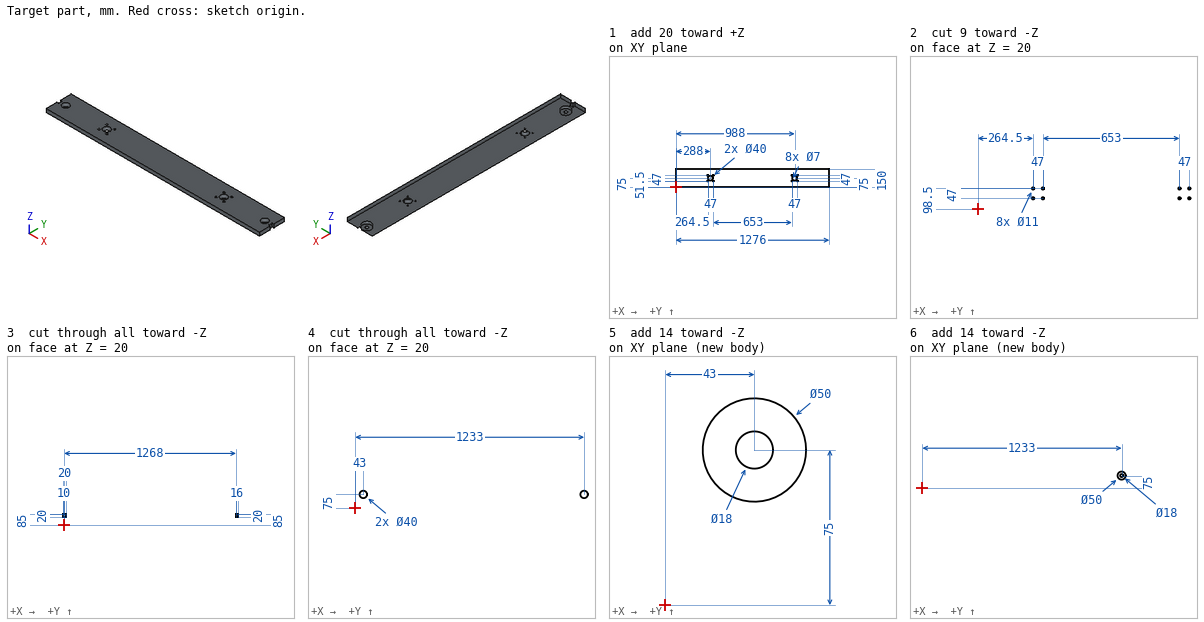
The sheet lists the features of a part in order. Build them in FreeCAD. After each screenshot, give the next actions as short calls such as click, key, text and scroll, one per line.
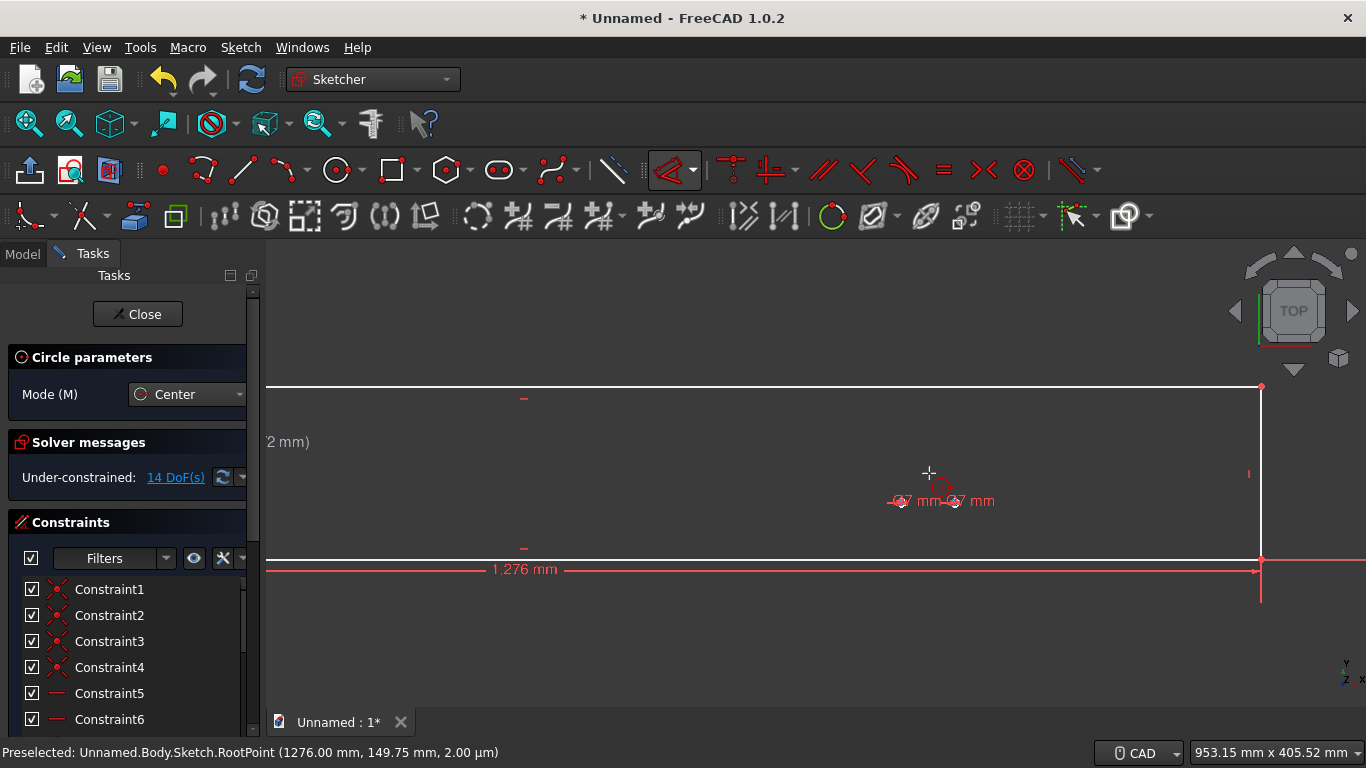
click(929, 473)
move(945, 457)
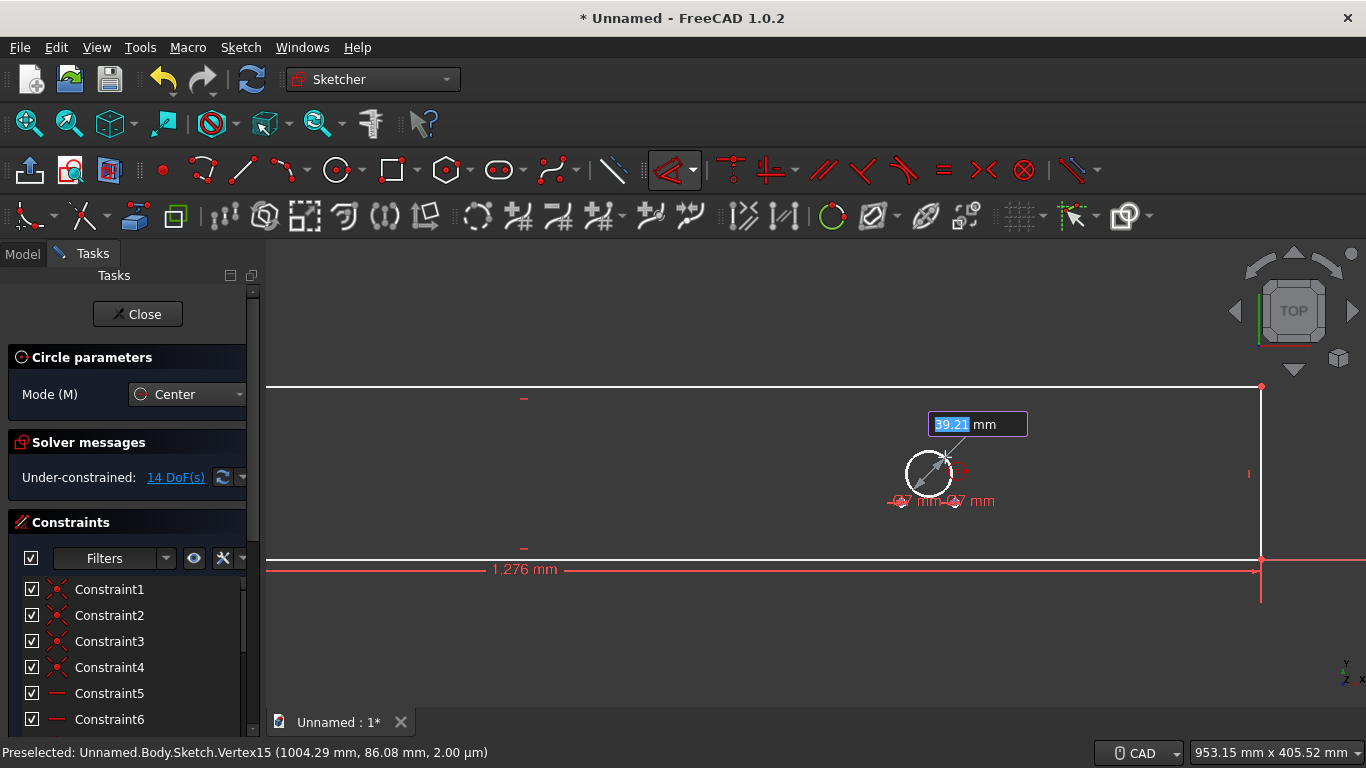
text(40)
key(Return)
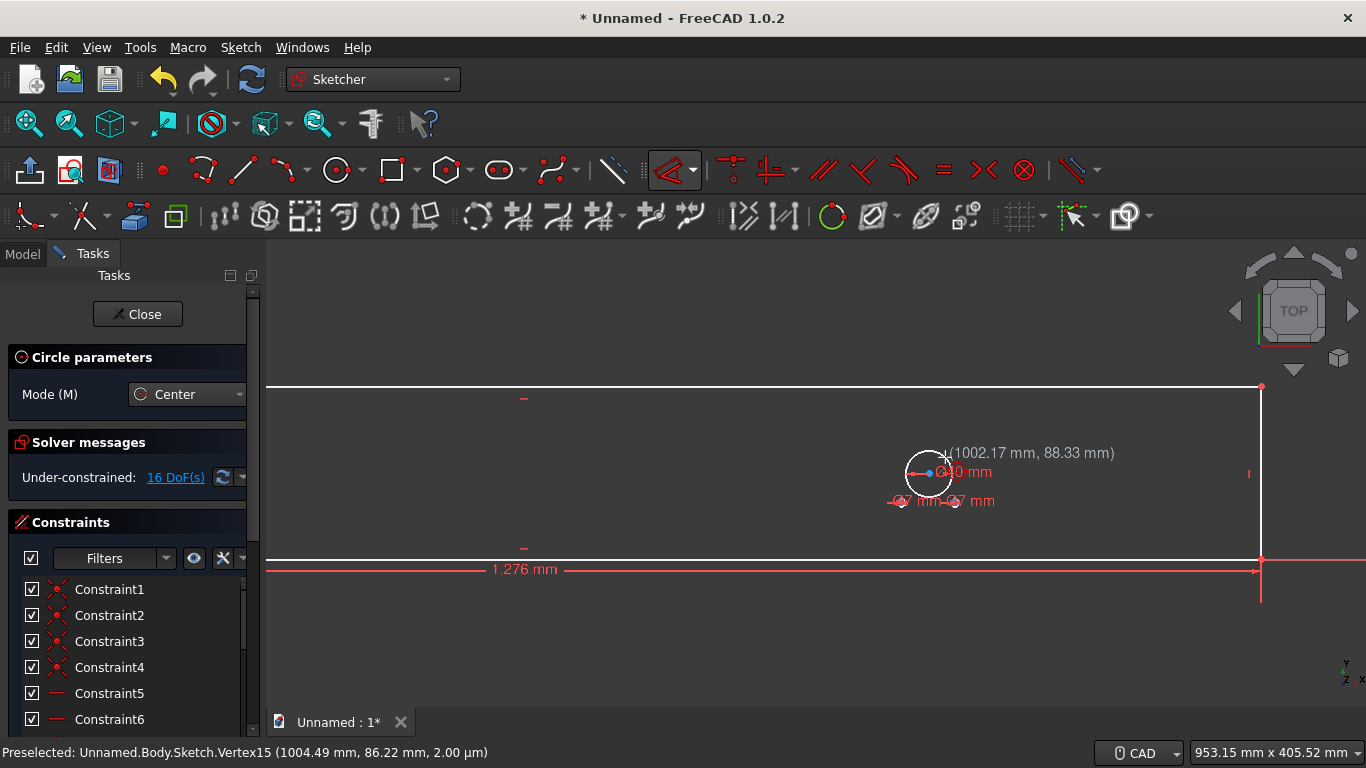
scroll(902, 446, up, 9)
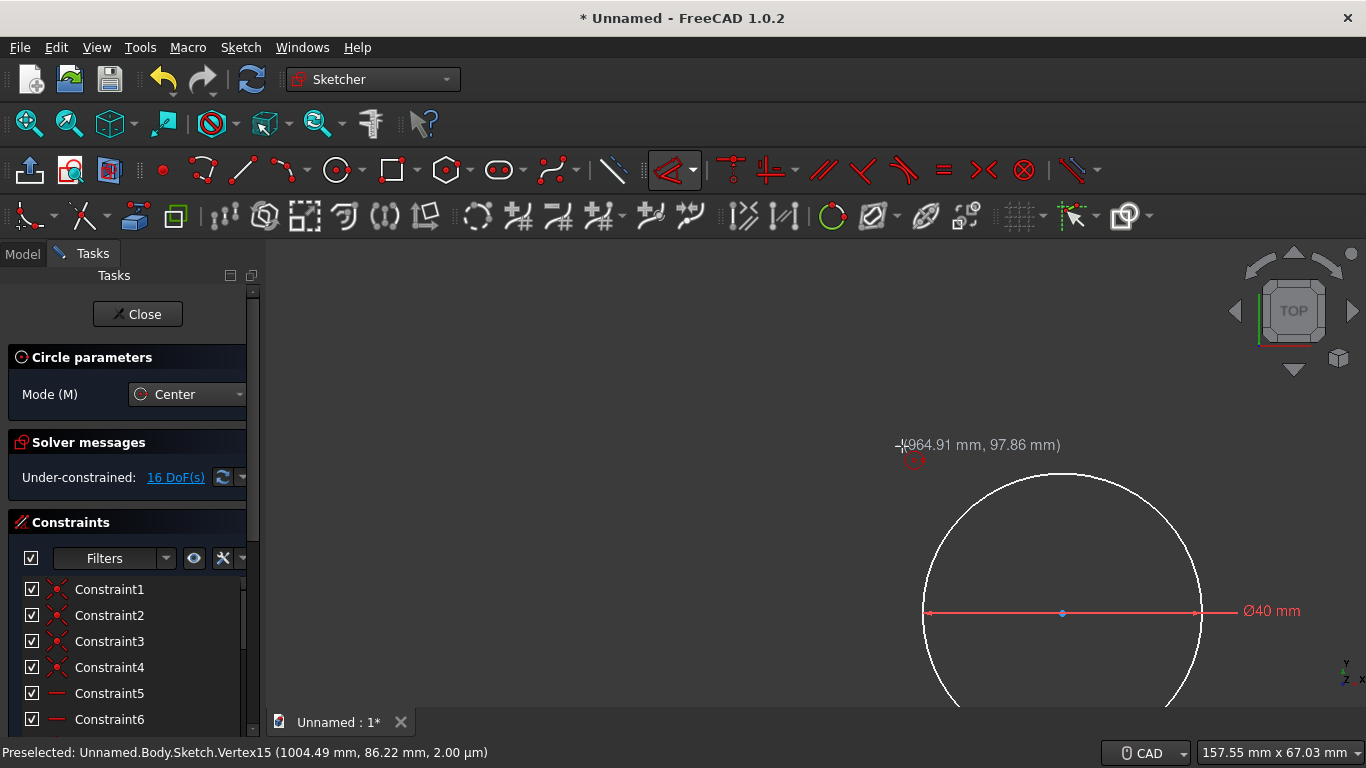
scroll(918, 462, down, 13)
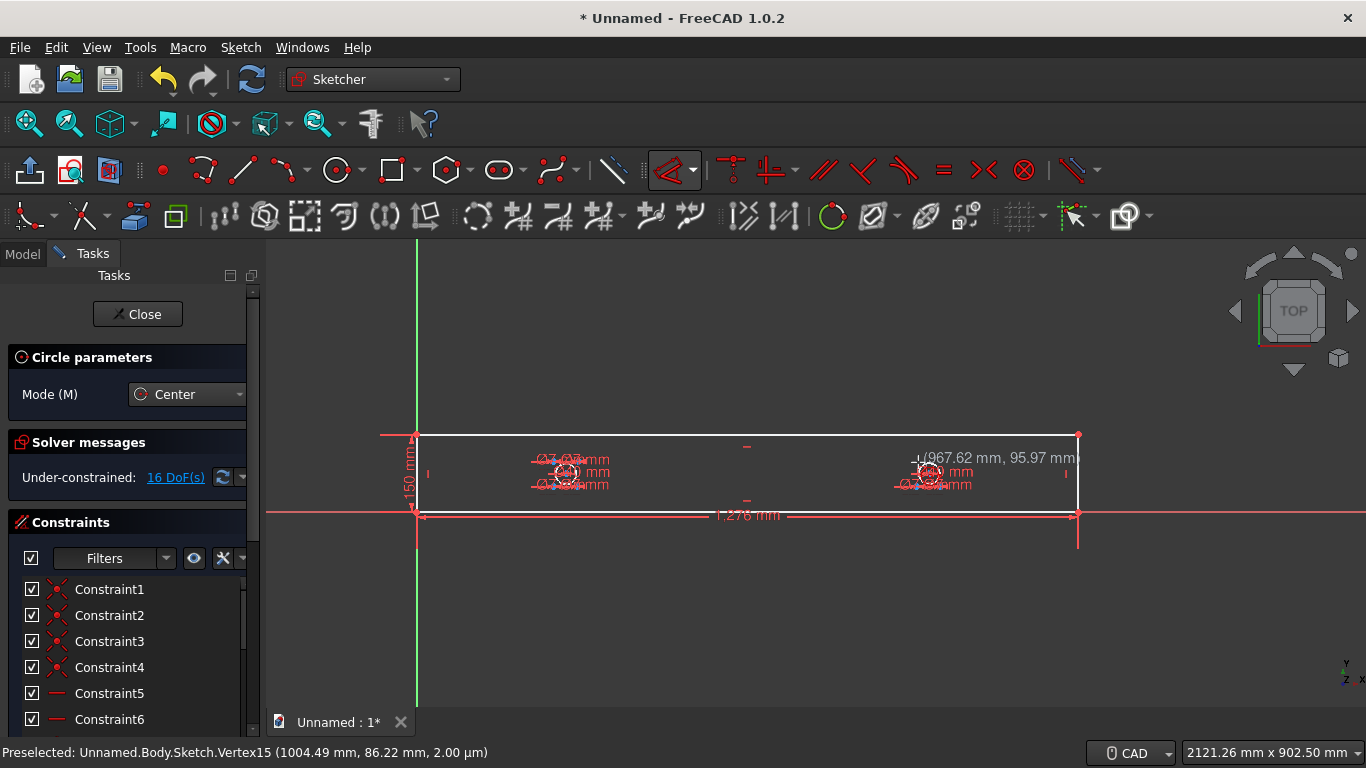
scroll(917, 461, up, 5)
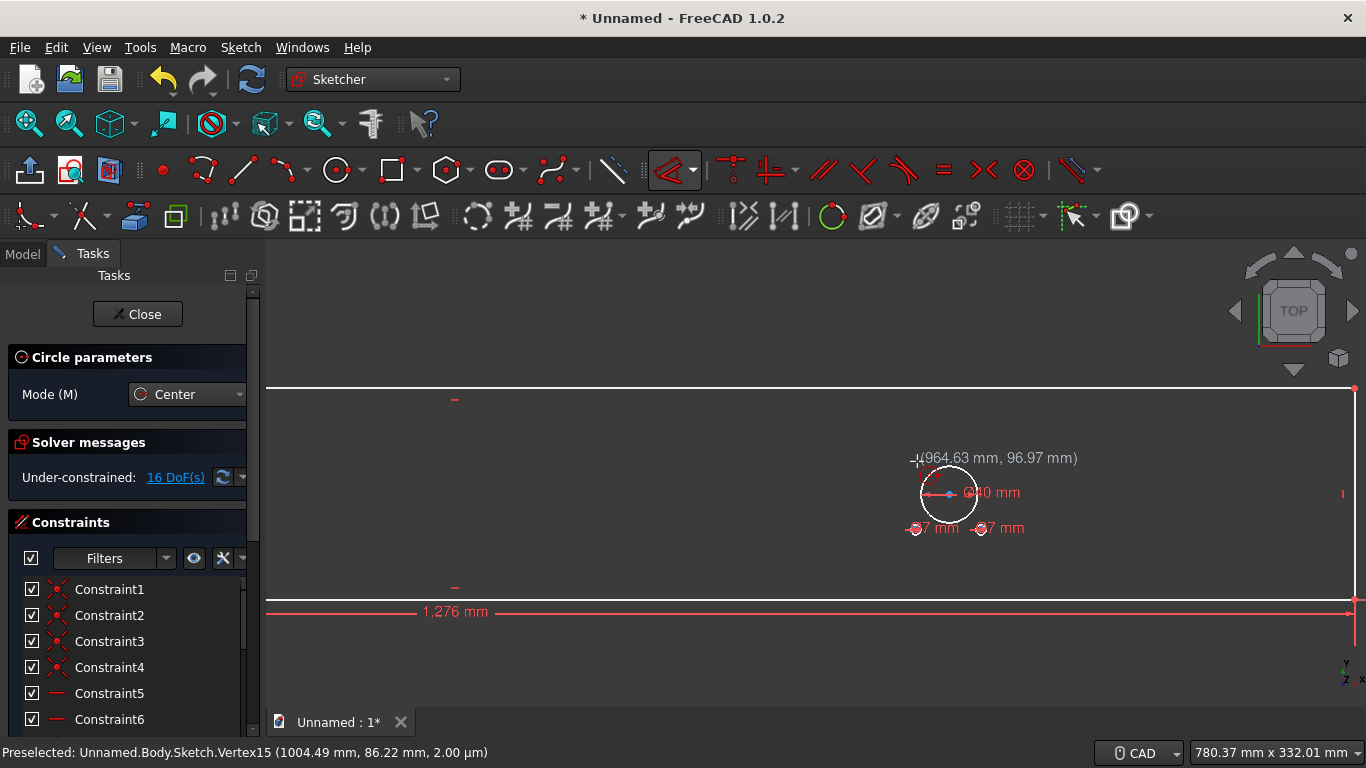
click(916, 461)
move(919, 457)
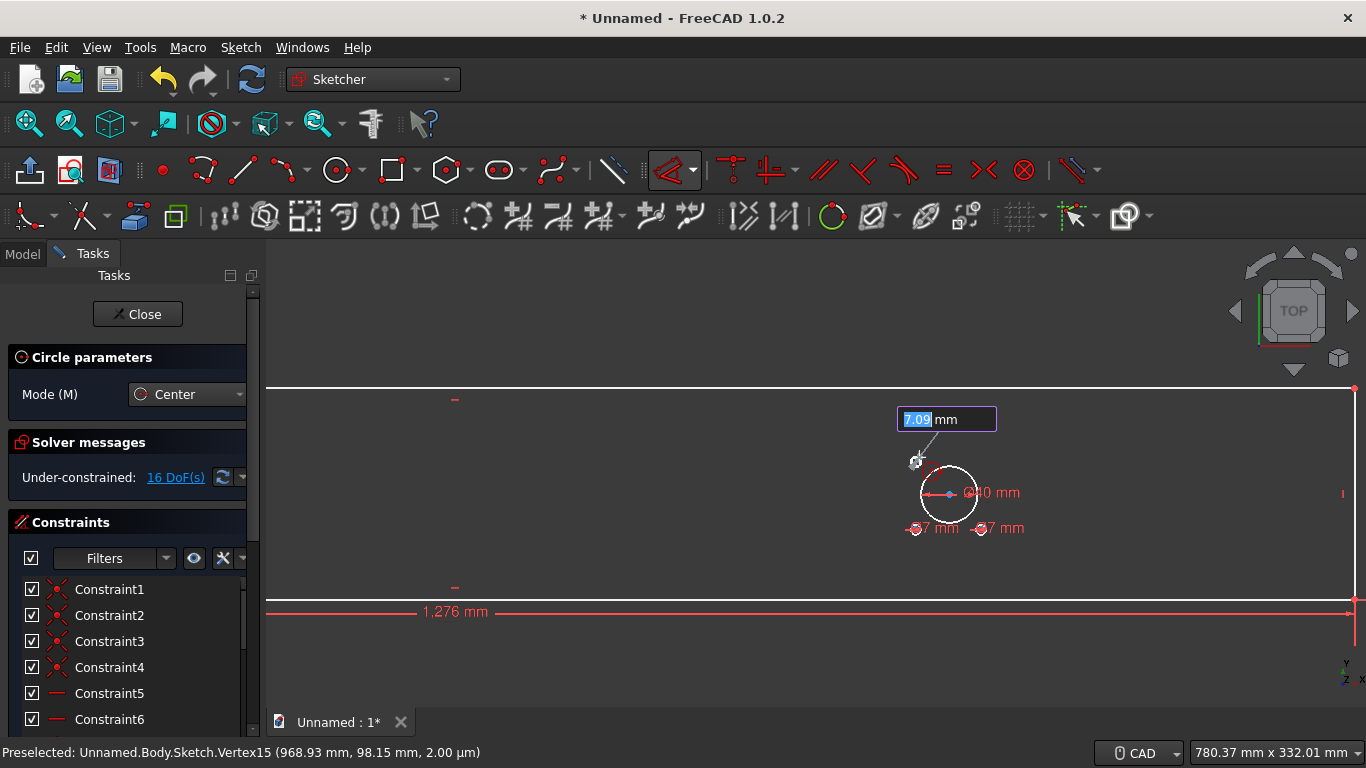
text(7)
key(Return)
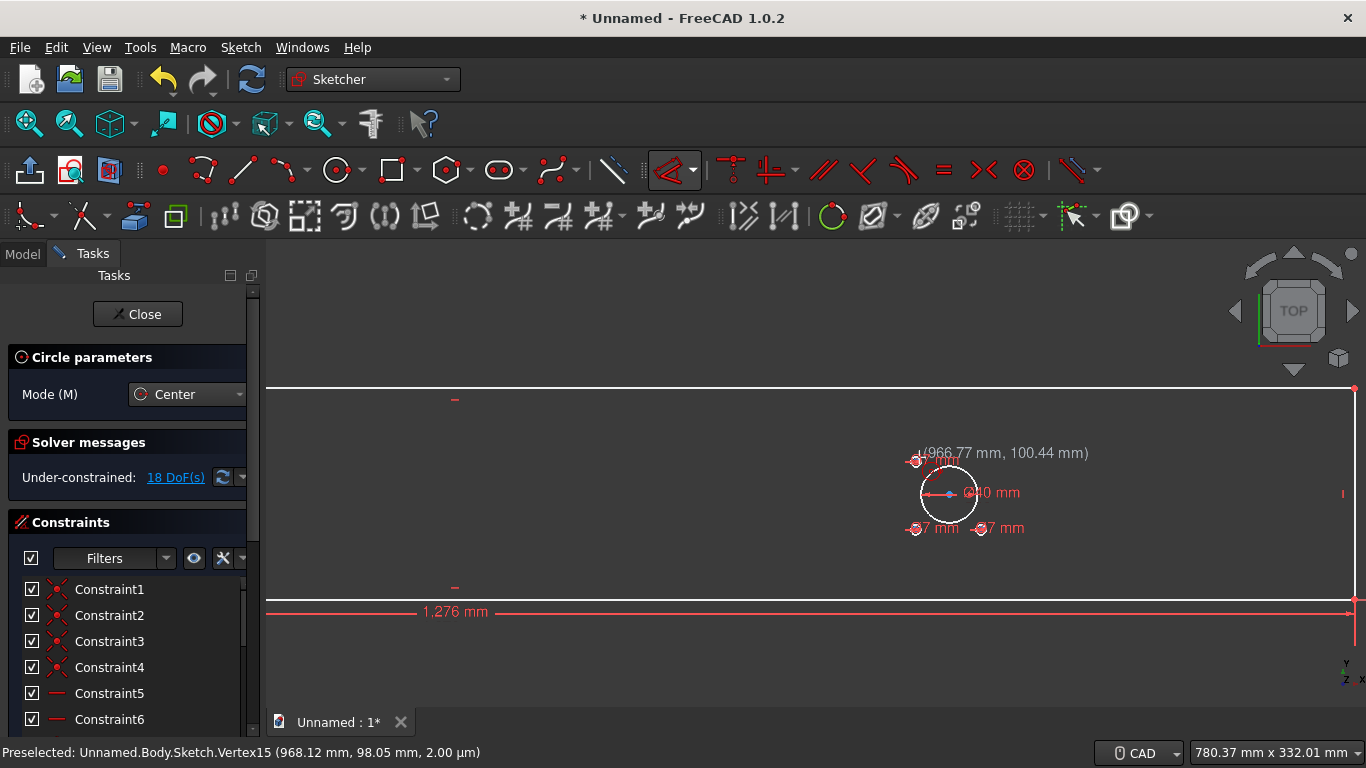
scroll(982, 461, up, 8)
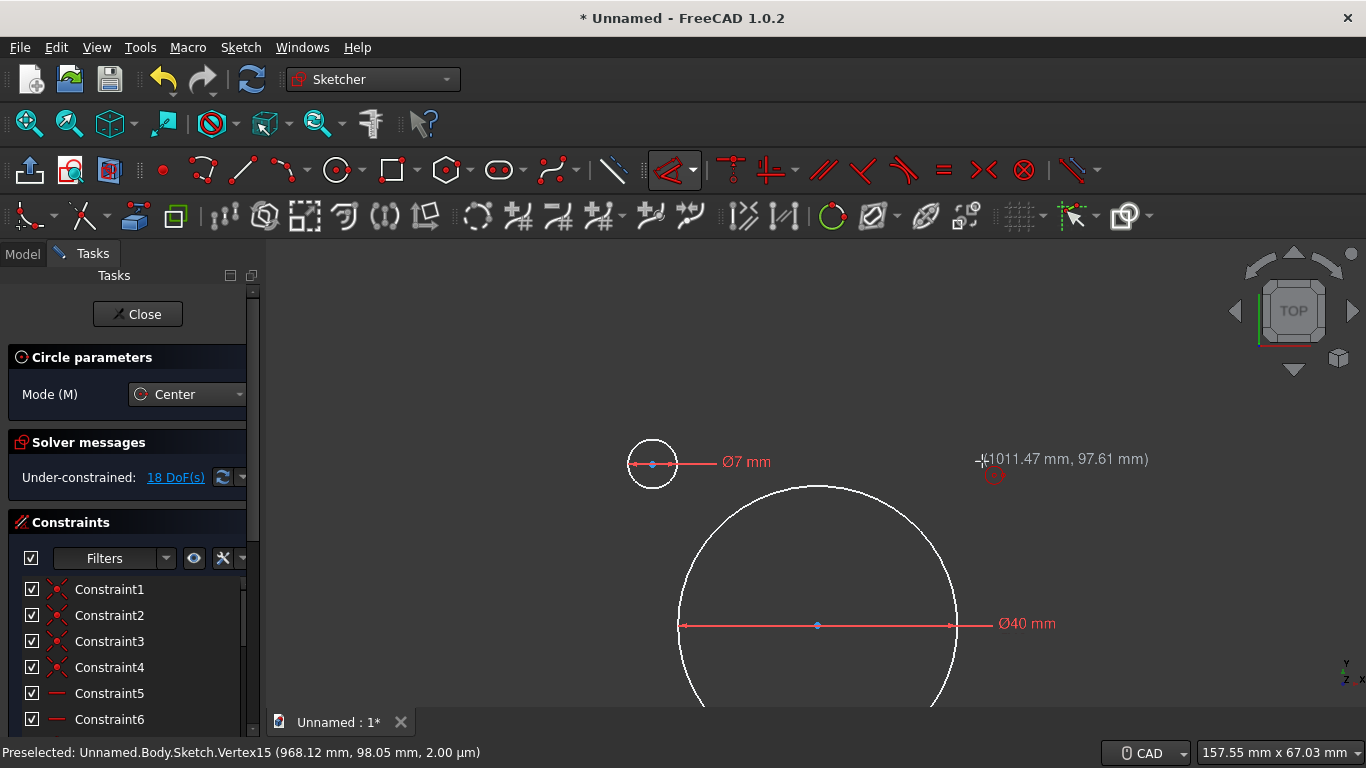
scroll(938, 461, down, 13)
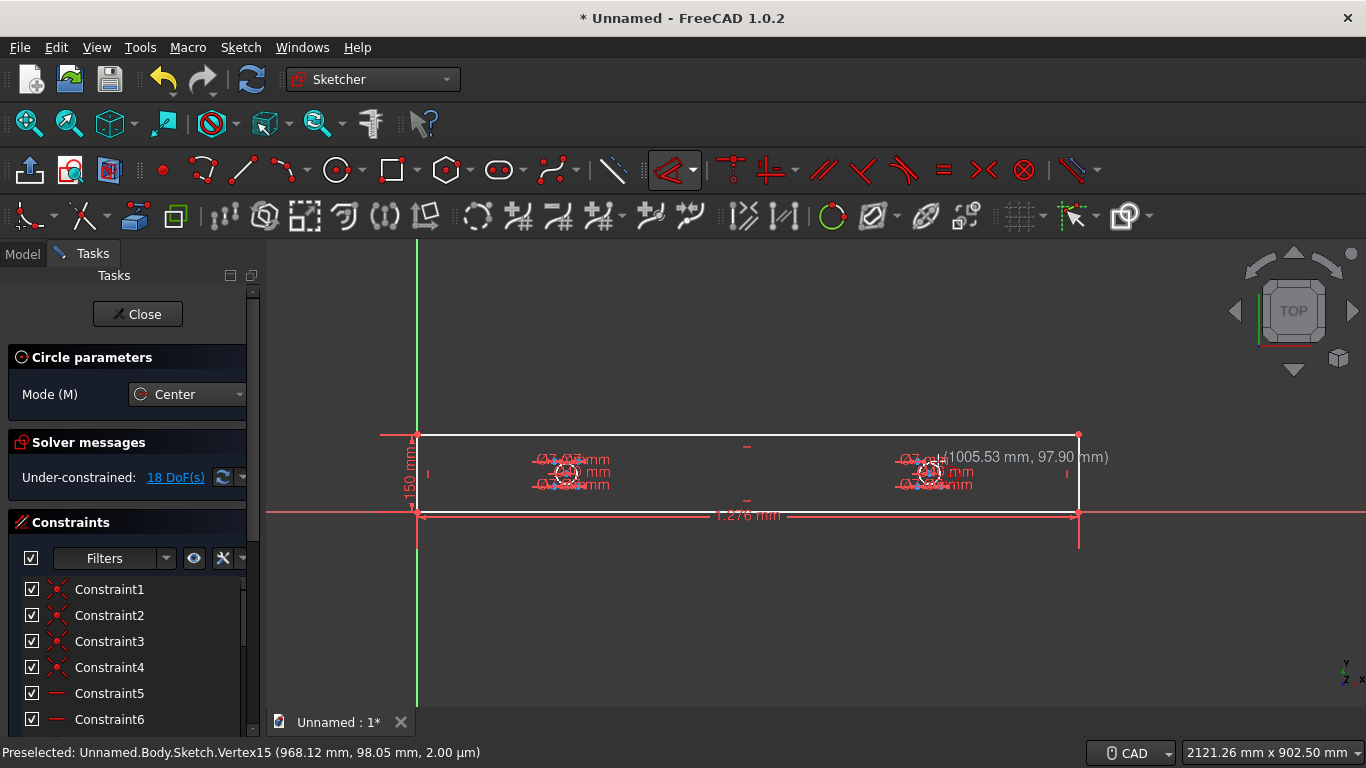
scroll(942, 461, up, 5)